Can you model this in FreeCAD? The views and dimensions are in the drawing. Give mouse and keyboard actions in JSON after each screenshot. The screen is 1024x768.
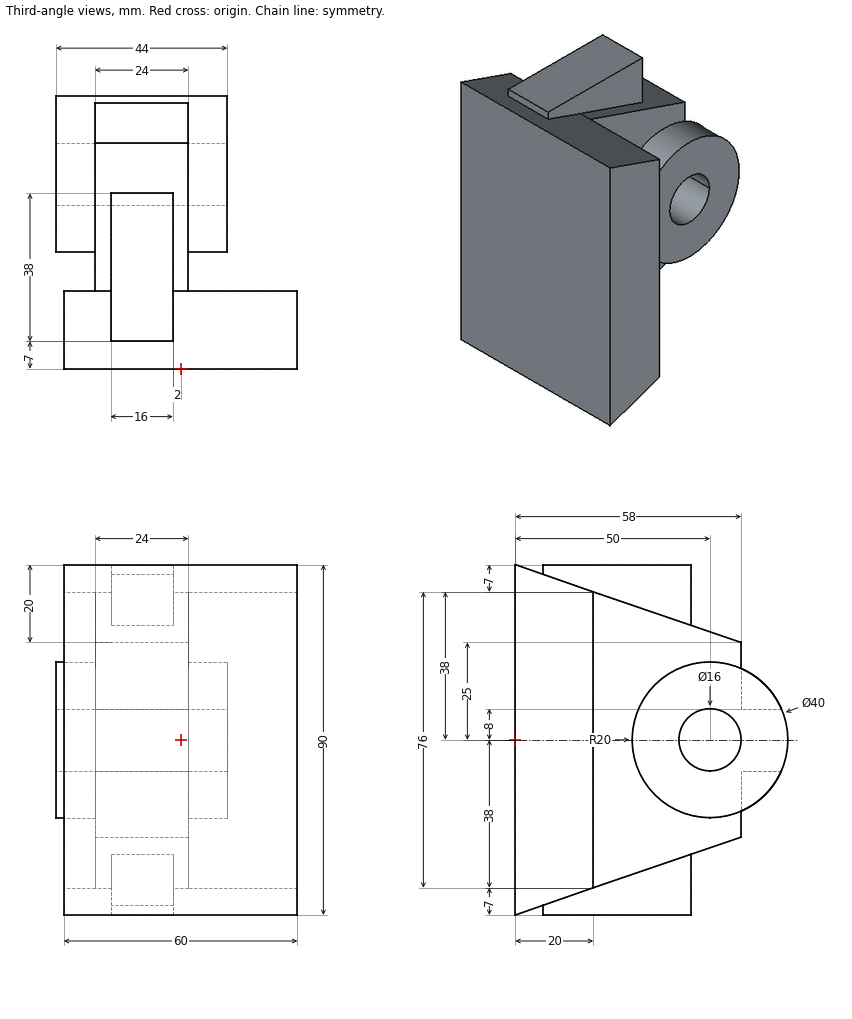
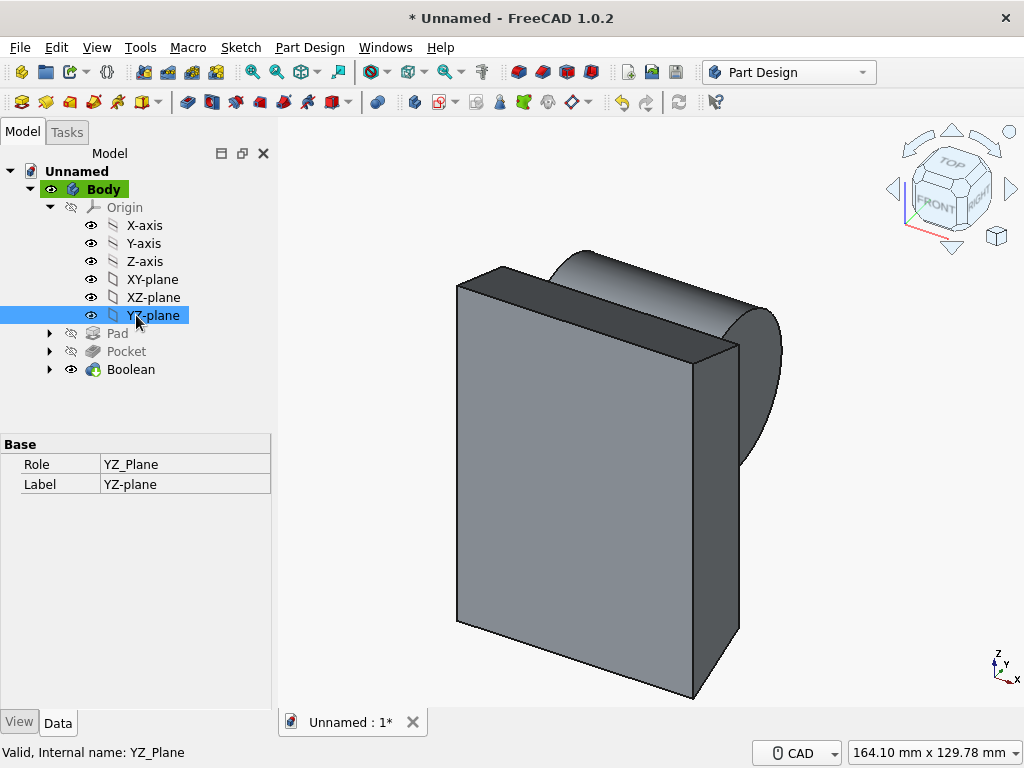
{"action": "left_click", "coordinate": [572, 102]}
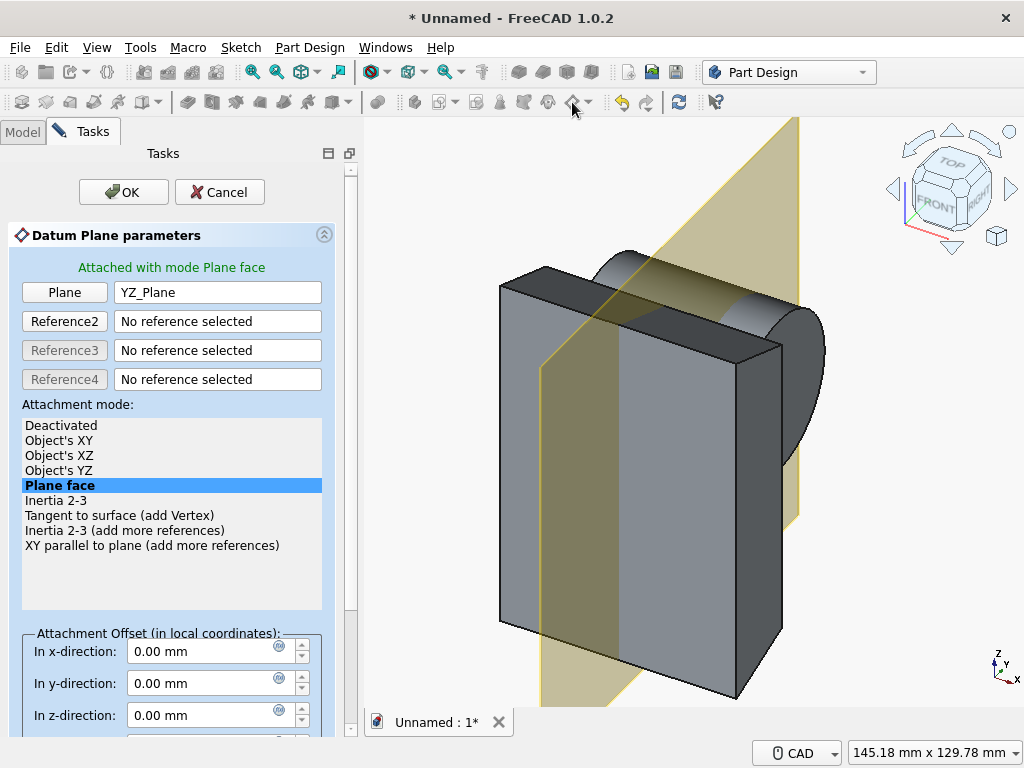
{"action": "triple_click", "coordinate": [210, 715]}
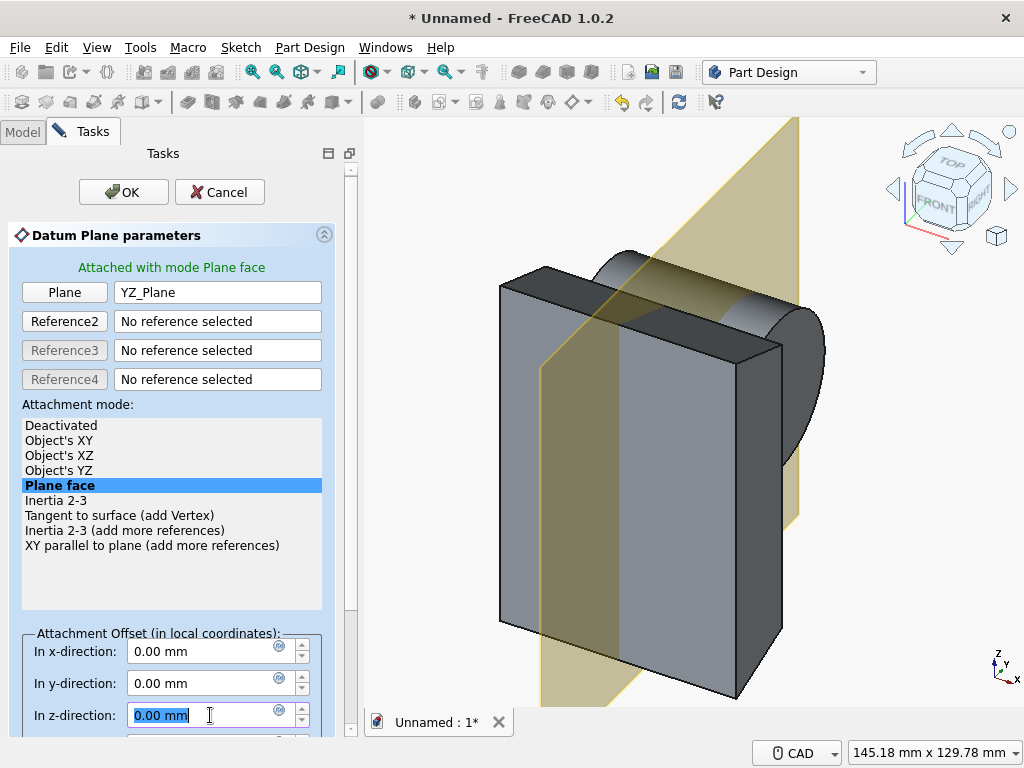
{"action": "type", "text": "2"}
{"action": "key", "text": "Tab"}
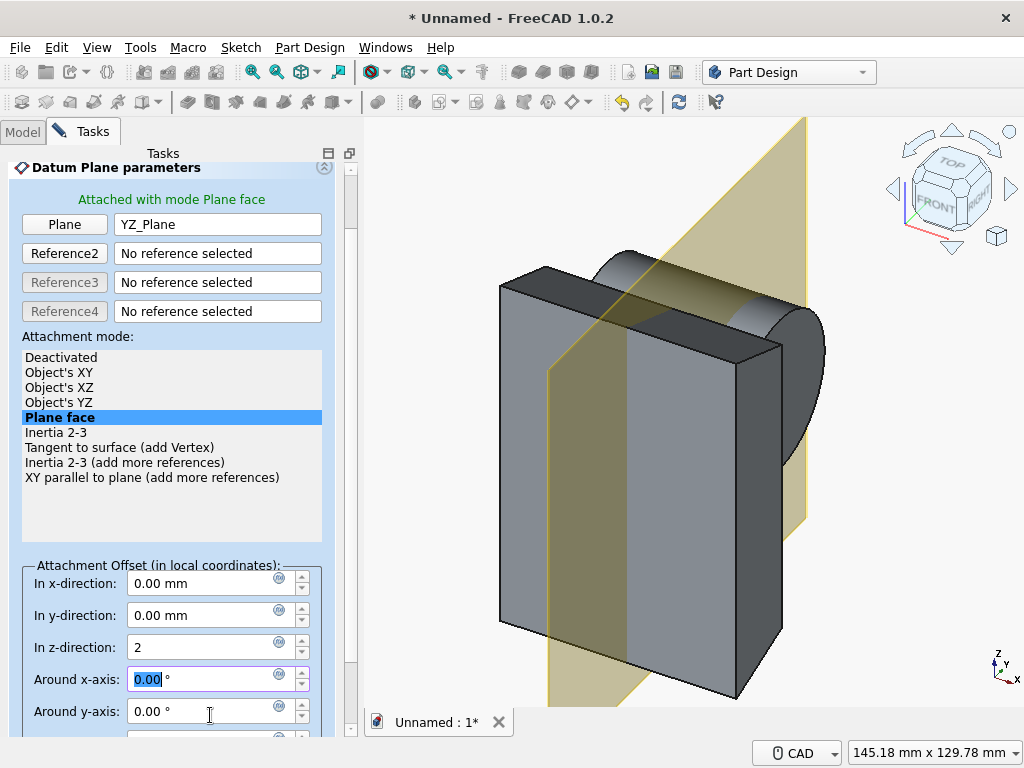
{"action": "scroll", "coordinate": [351, 450], "scroll_direction": "up", "scroll_amount": 2}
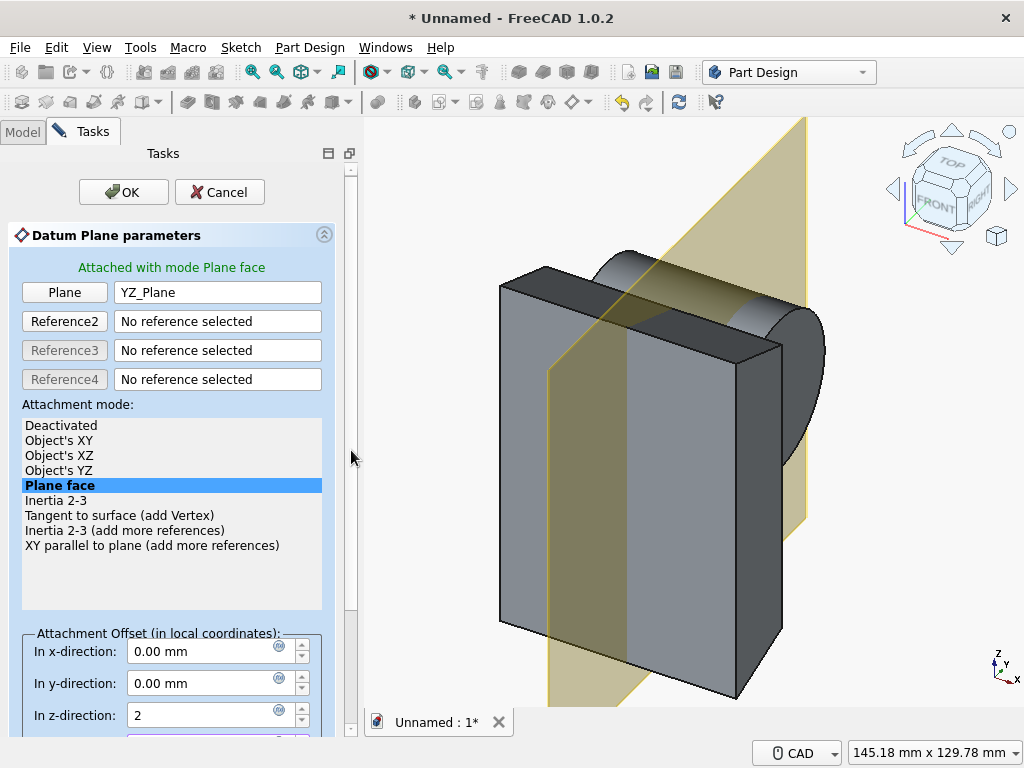
{"action": "left_click", "coordinate": [124, 192]}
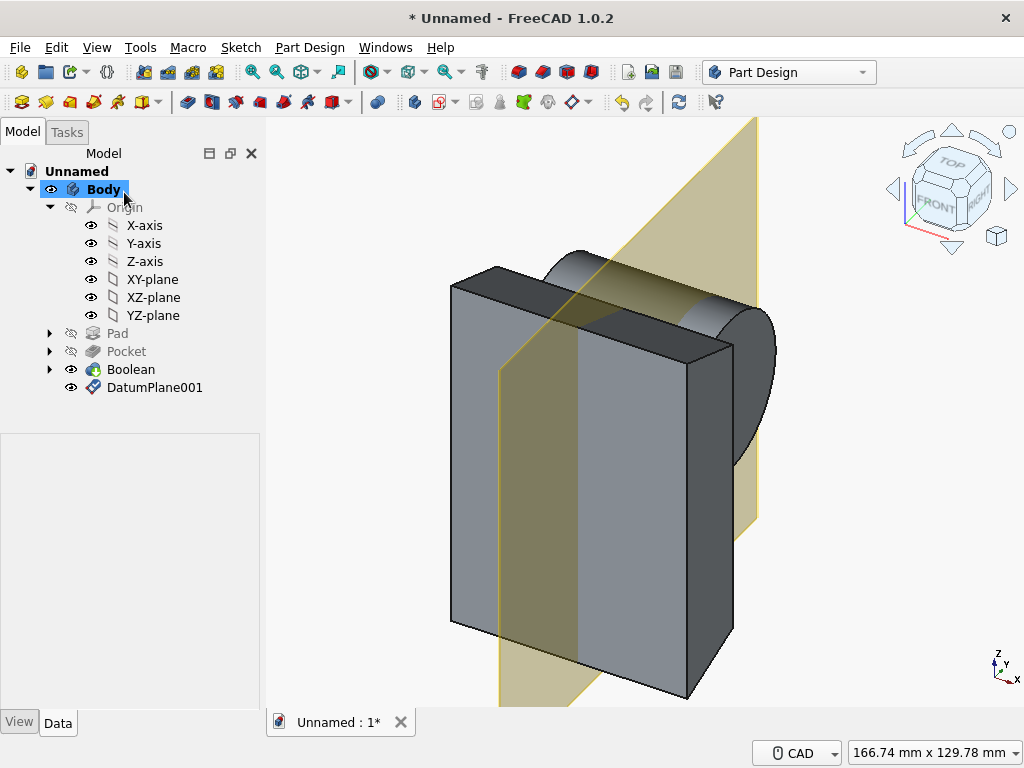
{"action": "left_click", "coordinate": [116, 387]}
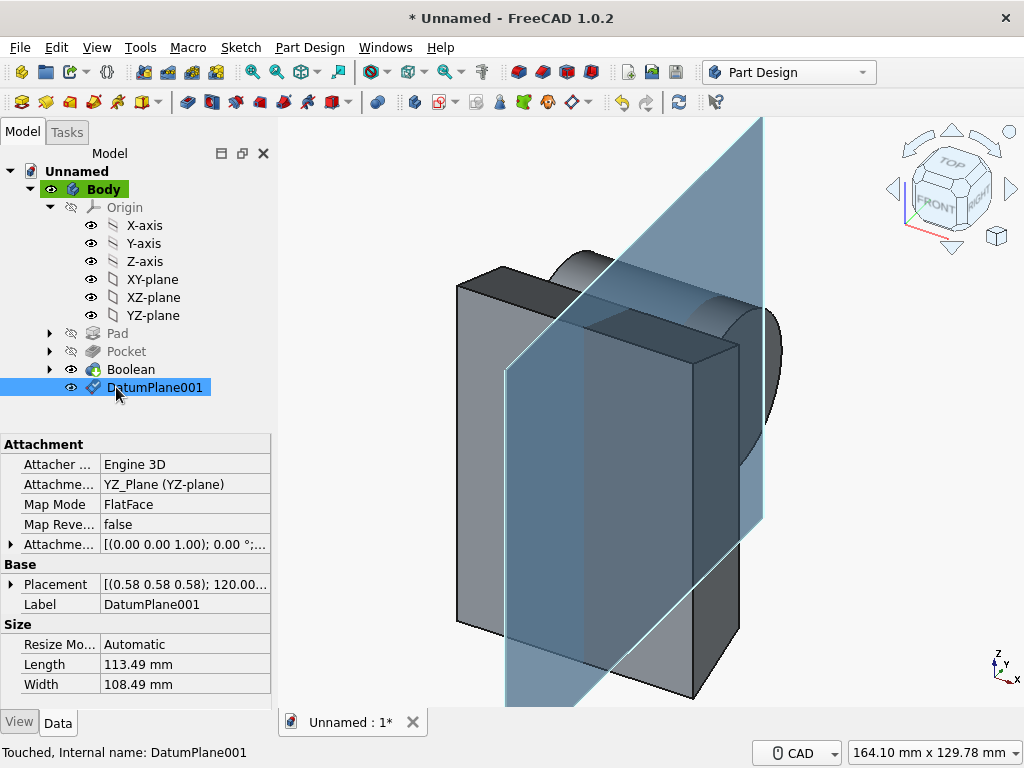
{"action": "left_click", "coordinate": [440, 102]}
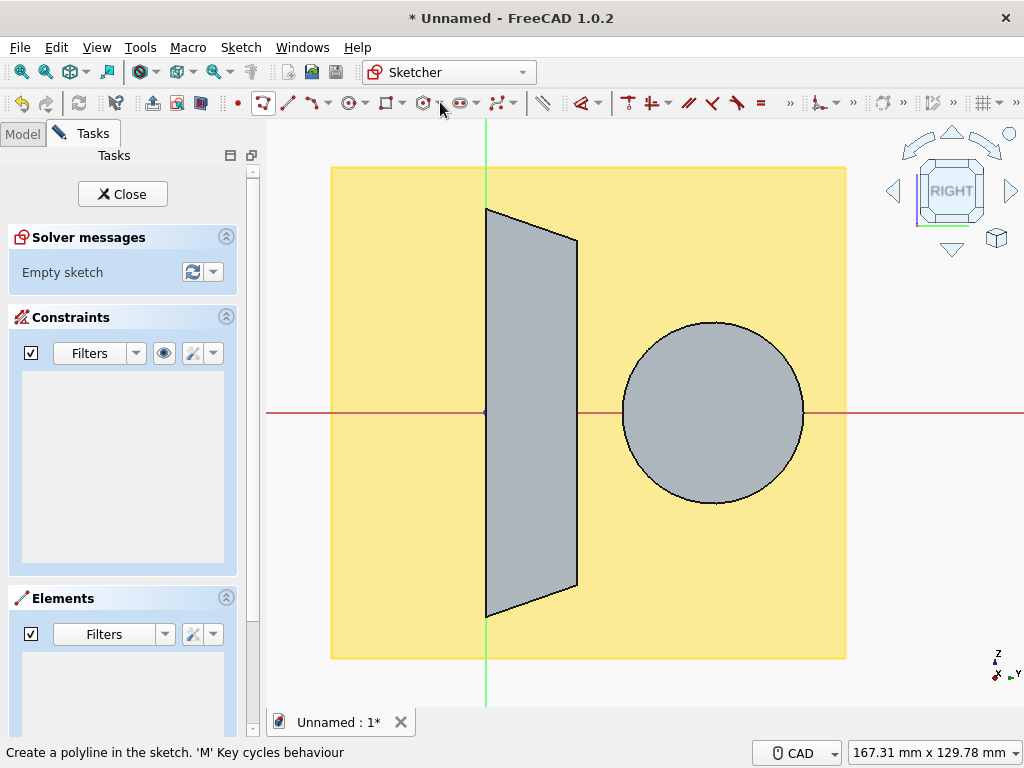
{"action": "left_click", "coordinate": [202, 104]}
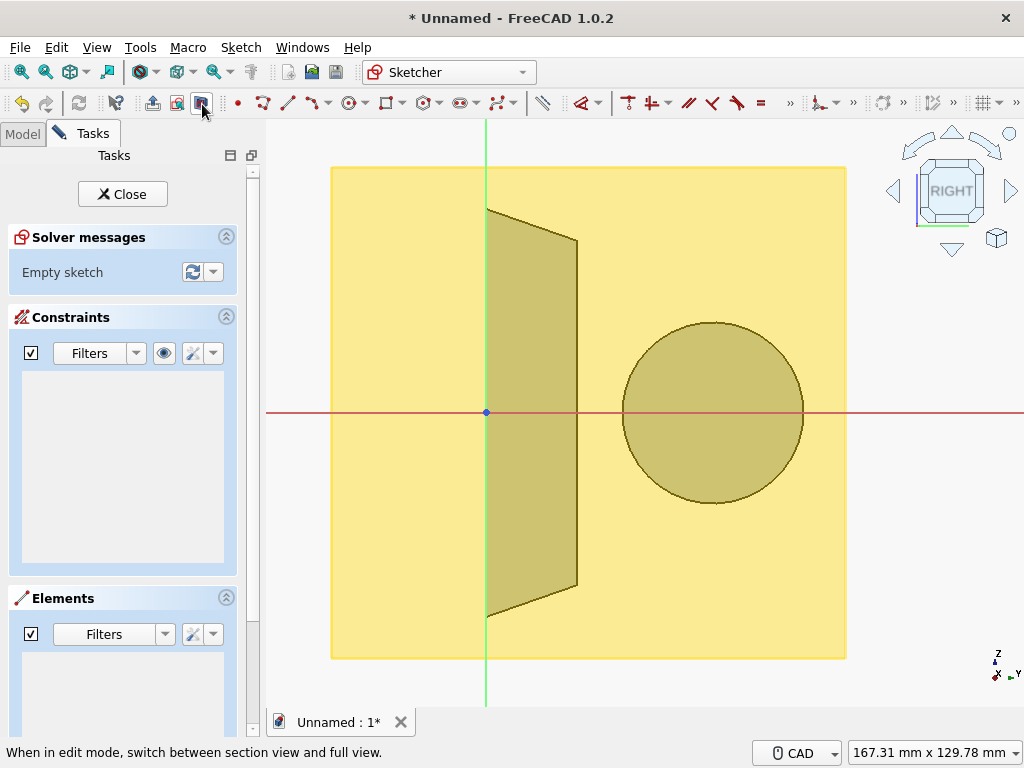
{"action": "key", "text": "g m"}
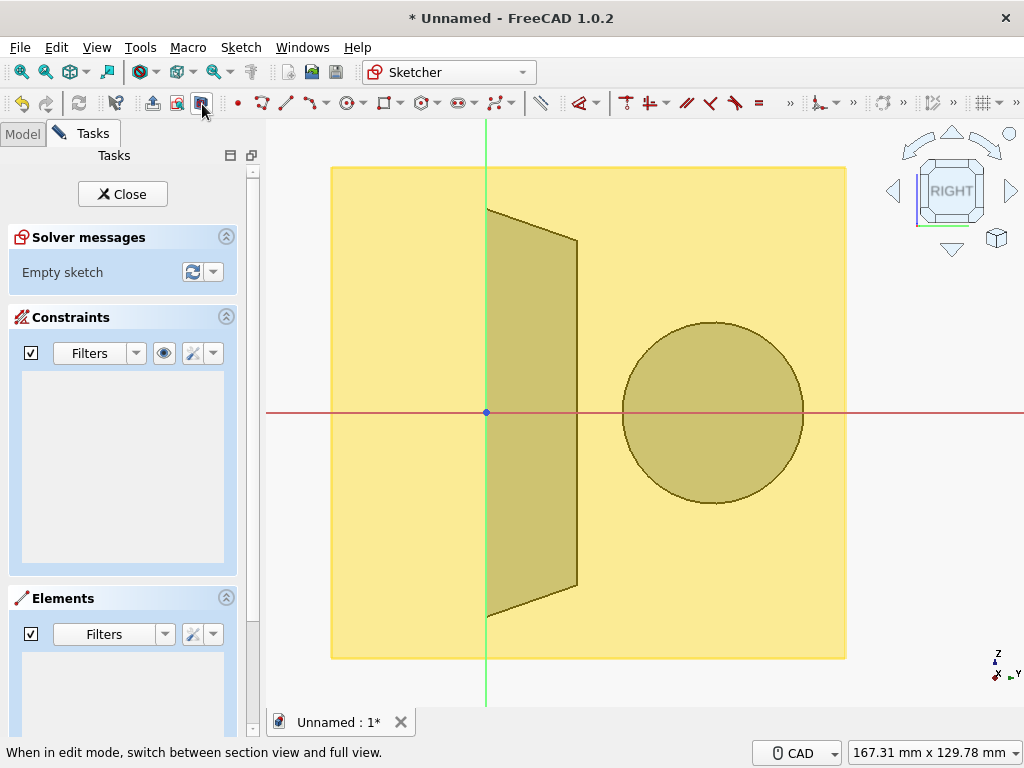
{"action": "left_click", "coordinate": [749, 330]}
{"action": "left_click", "coordinate": [749, 300]}
{"action": "left_click", "coordinate": [577, 241]}
{"action": "left_click", "coordinate": [577, 585]}
{"action": "left_click", "coordinate": [749, 526]}
{"action": "left_click", "coordinate": [749, 496]}
{"action": "right_click", "coordinate": [749, 496]}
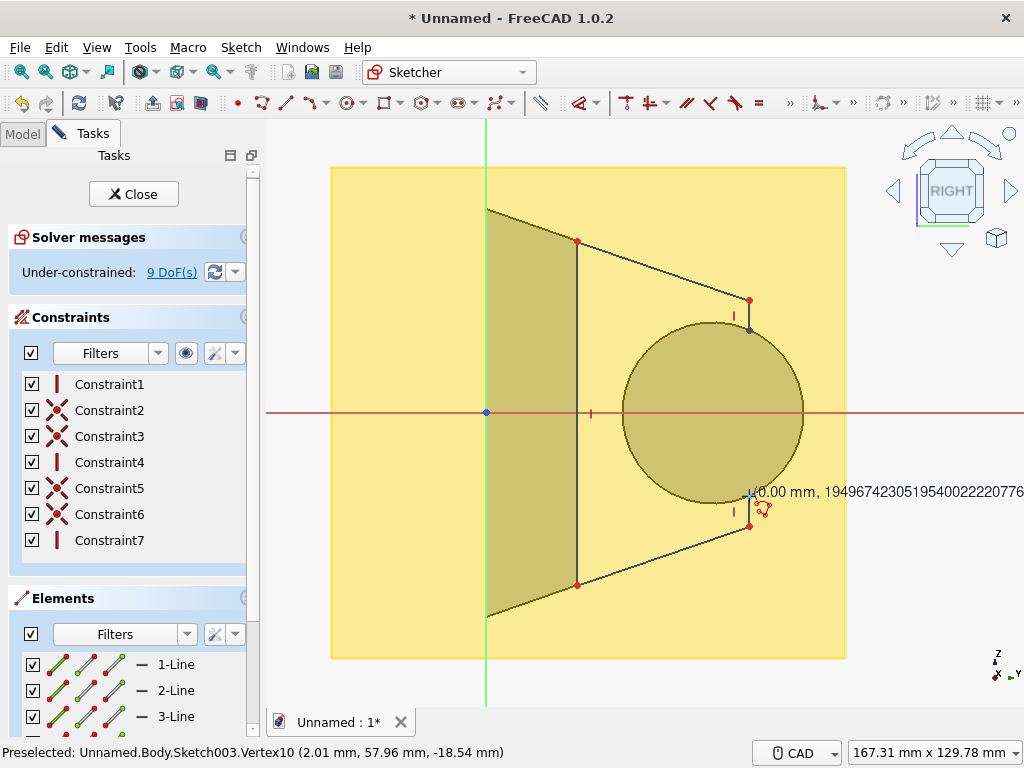
{"action": "left_click", "coordinate": [310, 104]}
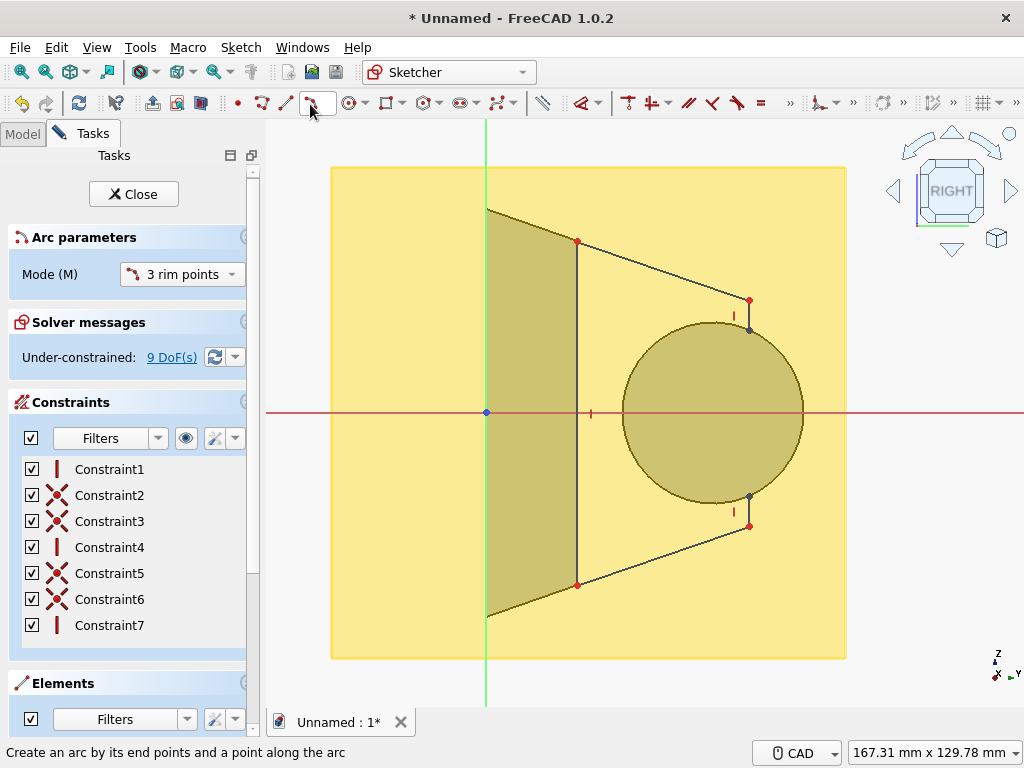
{"action": "left_click", "coordinate": [749, 497]}
{"action": "left_click", "coordinate": [749, 331]}
{"action": "left_click", "coordinate": [629, 378]}
{"action": "key", "text": "Escape"}